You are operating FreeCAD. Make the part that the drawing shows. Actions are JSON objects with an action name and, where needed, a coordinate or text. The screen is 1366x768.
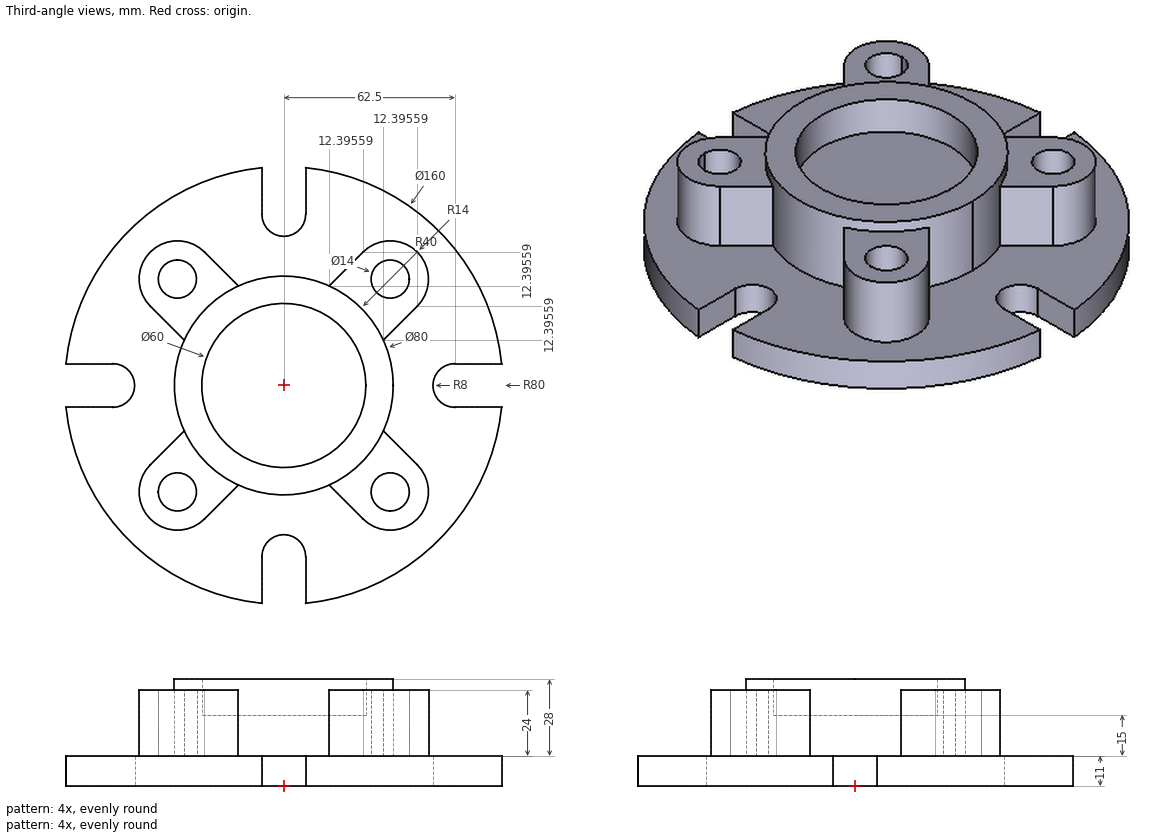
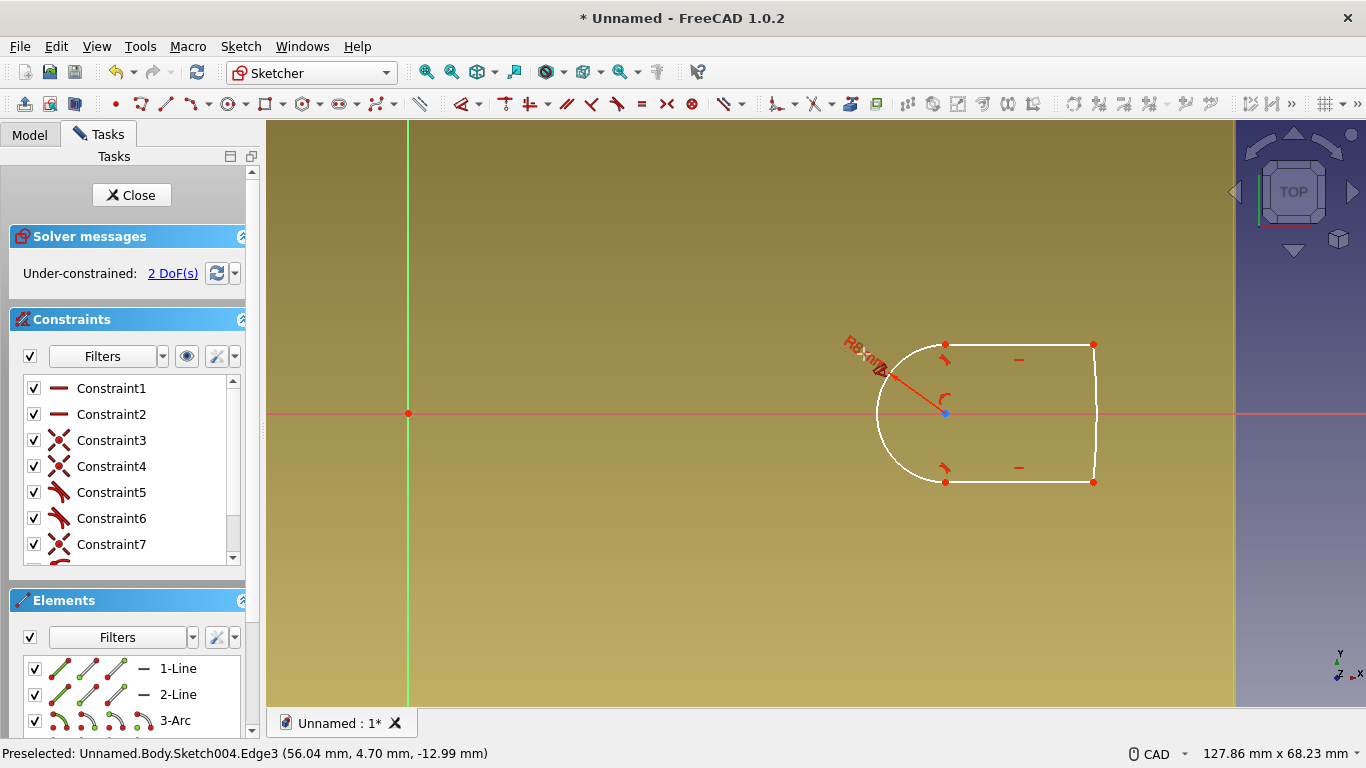
{"action": "left_click", "coordinate": [1096, 441]}
{"action": "left_click", "coordinate": [1128, 442]}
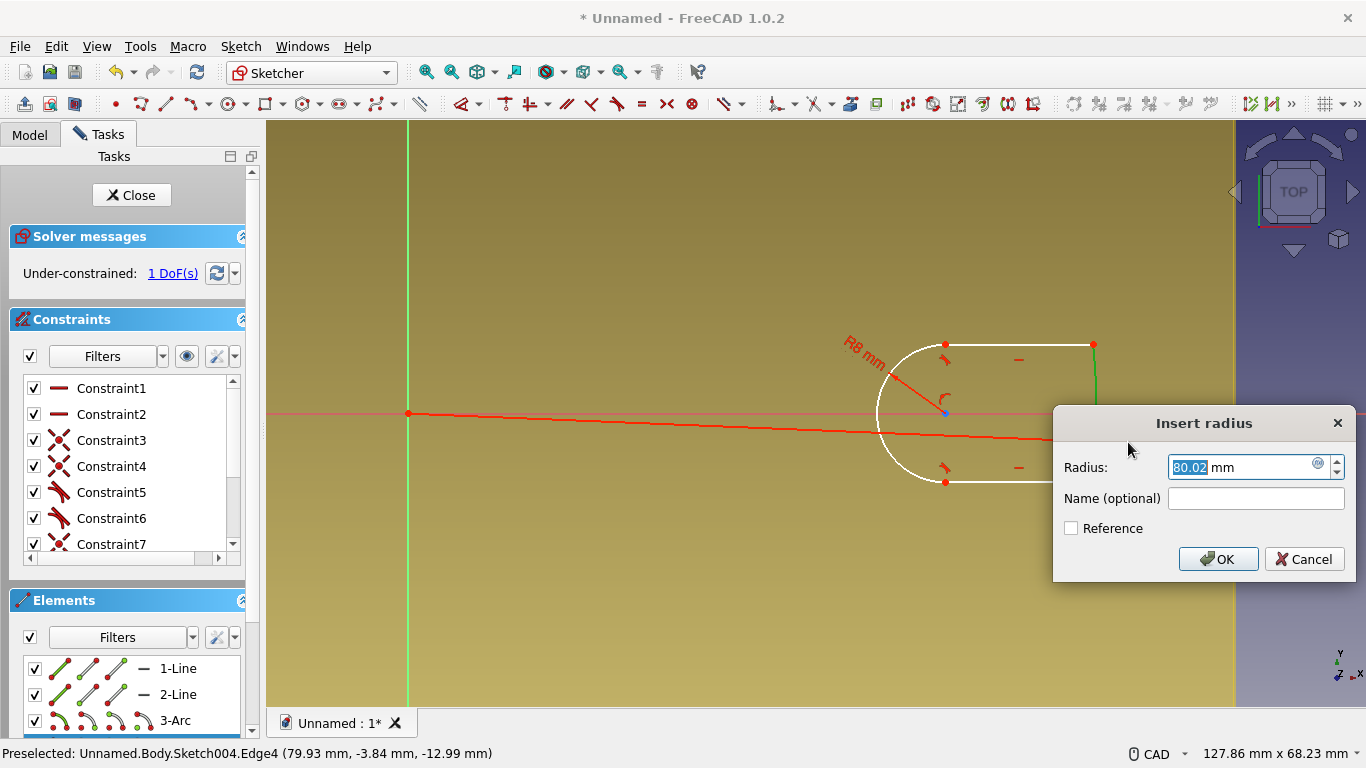
{"action": "type", "text": "80"}
{"action": "key", "text": "Return"}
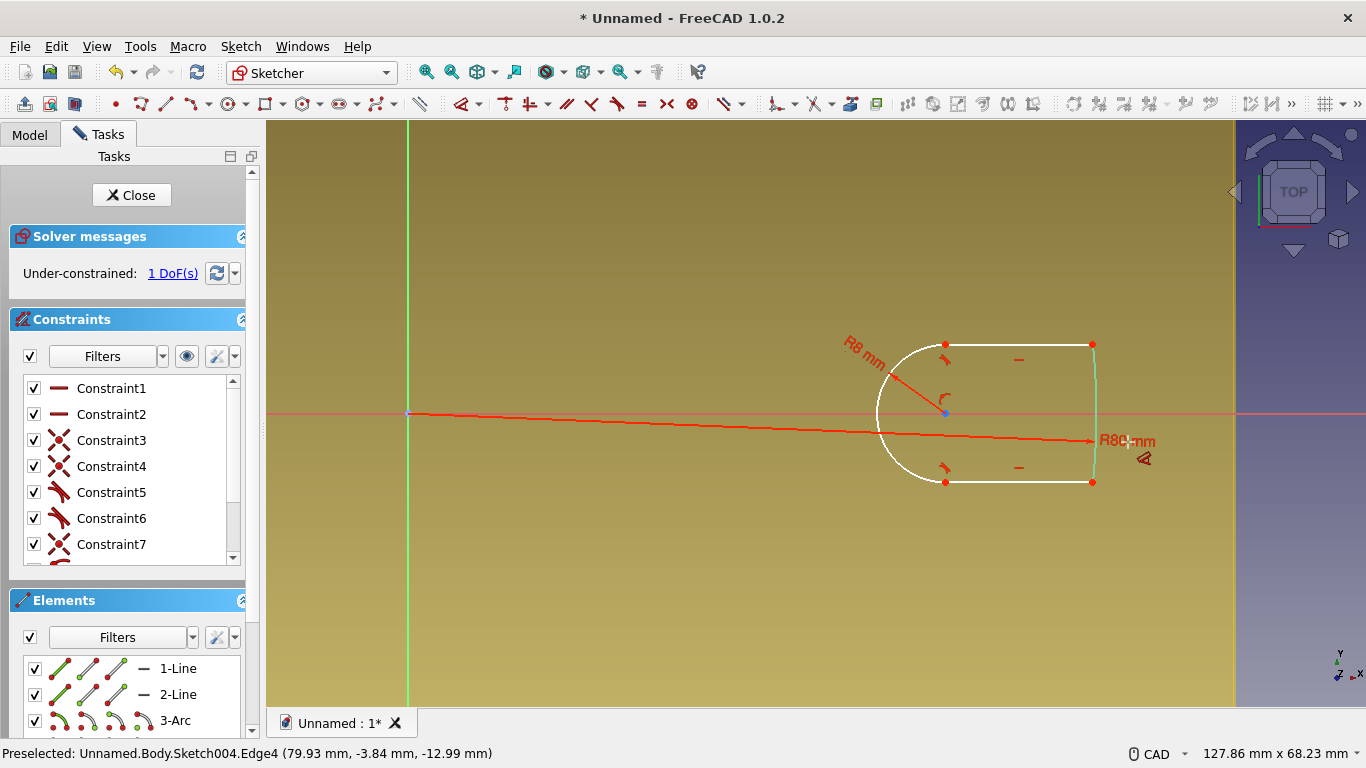
{"action": "left_click", "coordinate": [946, 345]}
{"action": "left_click", "coordinate": [677, 311]}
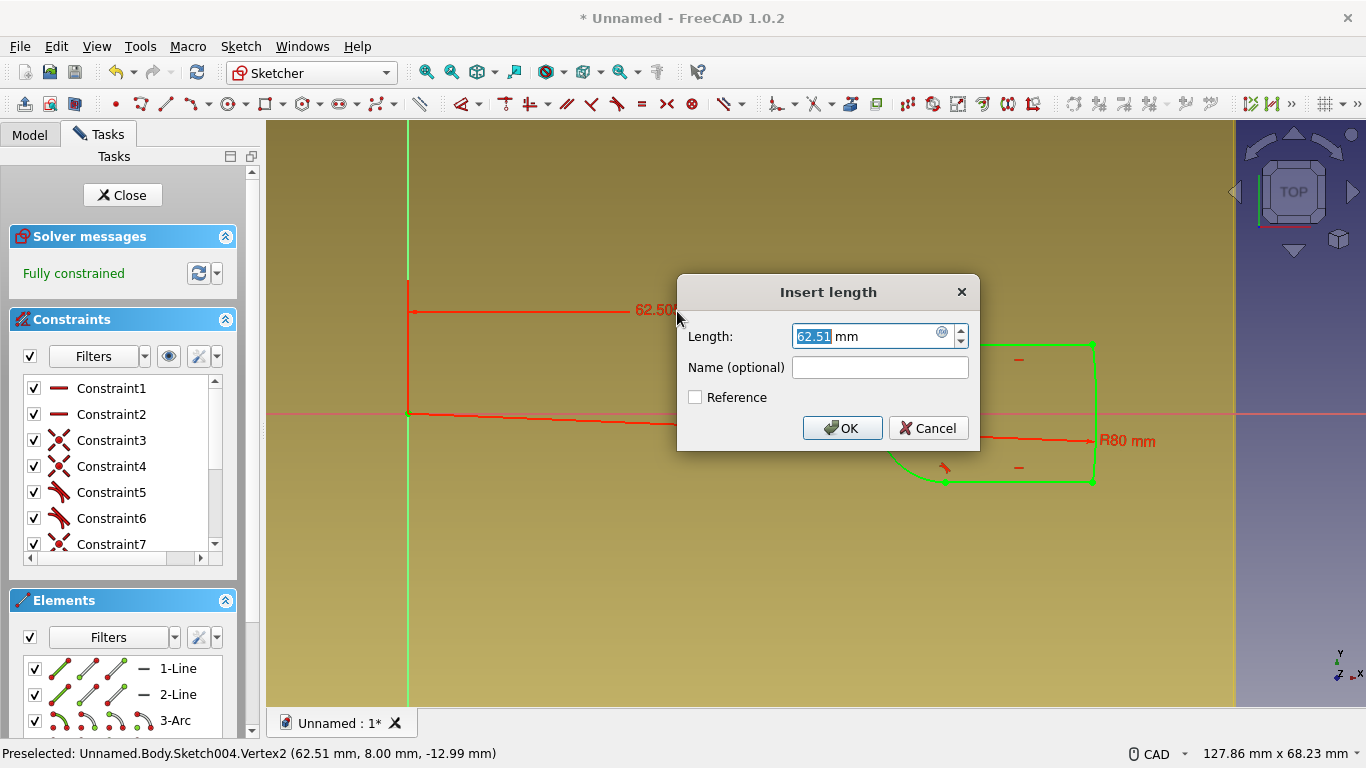
{"action": "type", "text": "62.5"}
{"action": "key", "text": "Return"}
{"action": "key", "text": "Escape"}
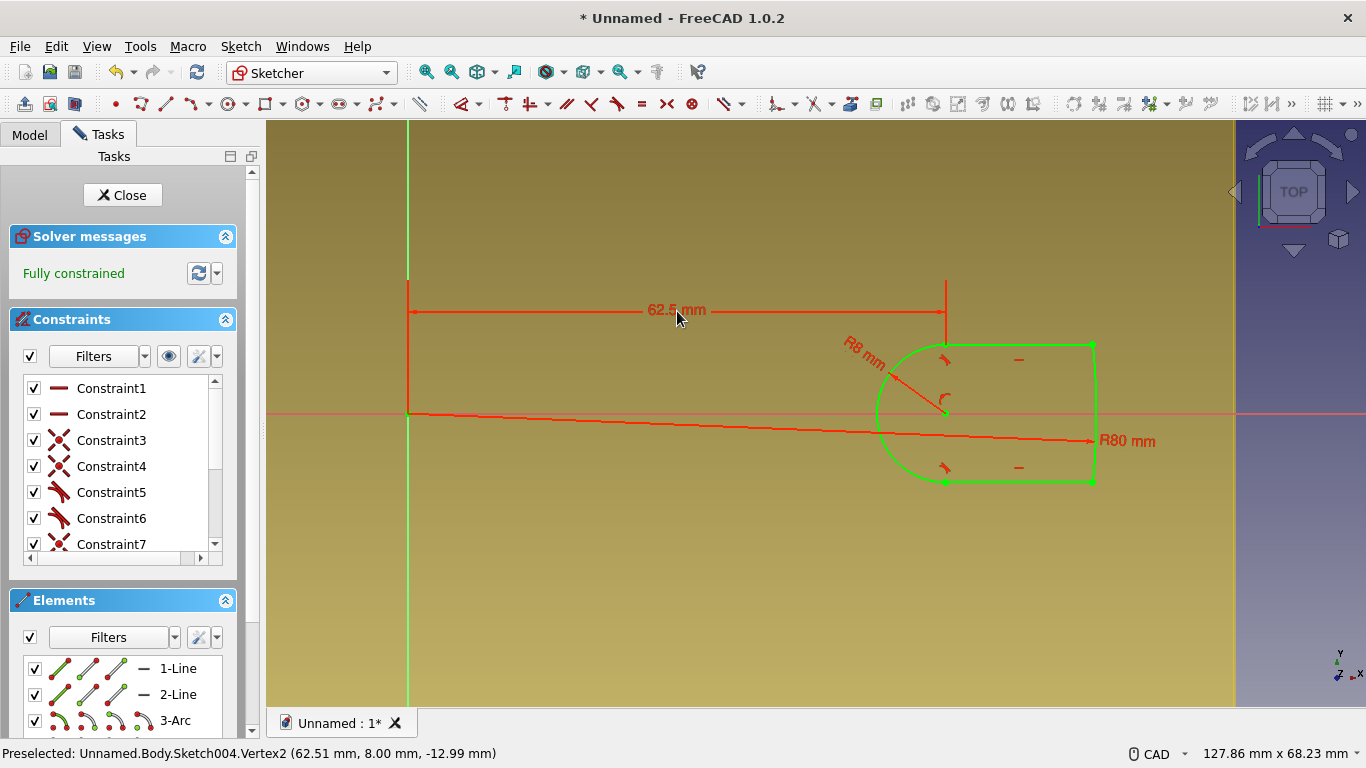
{"action": "left_click", "coordinate": [123, 195]}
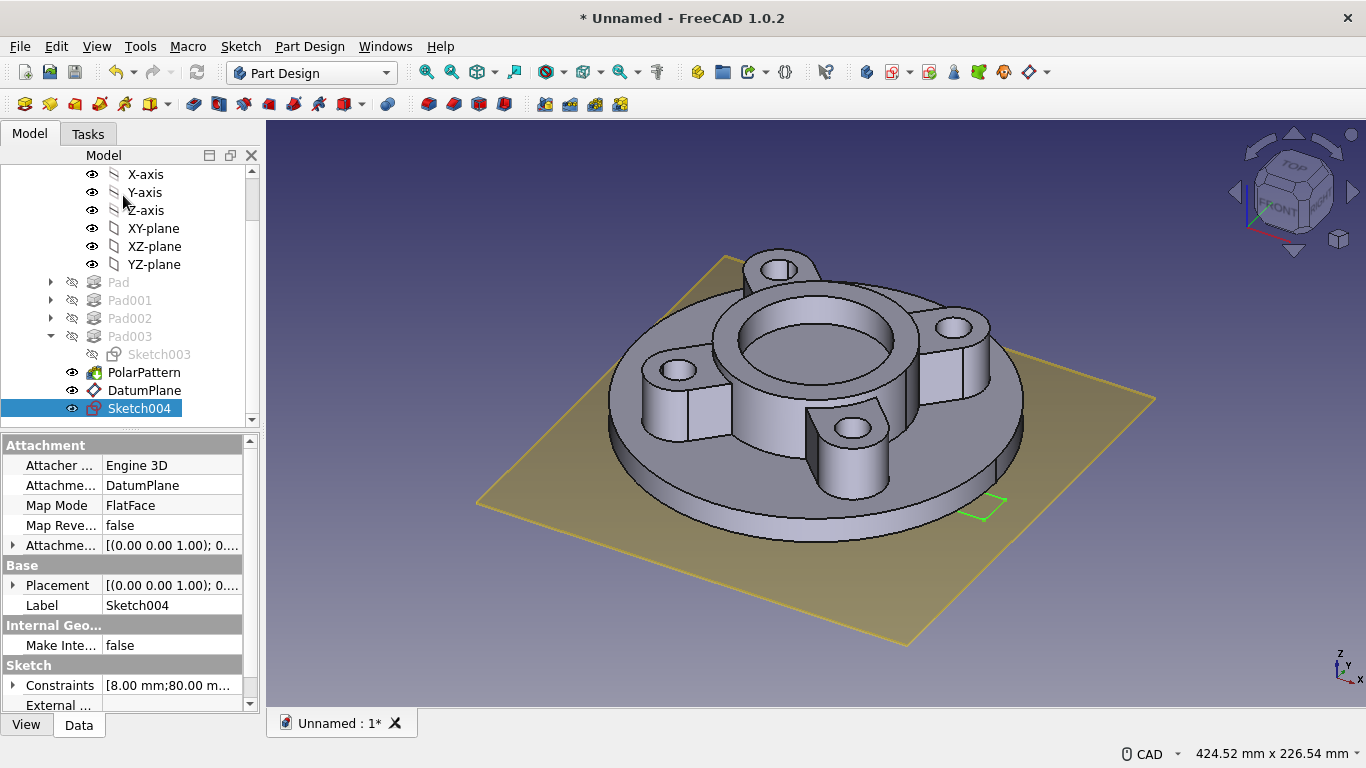
{"action": "left_click", "coordinate": [194, 104]}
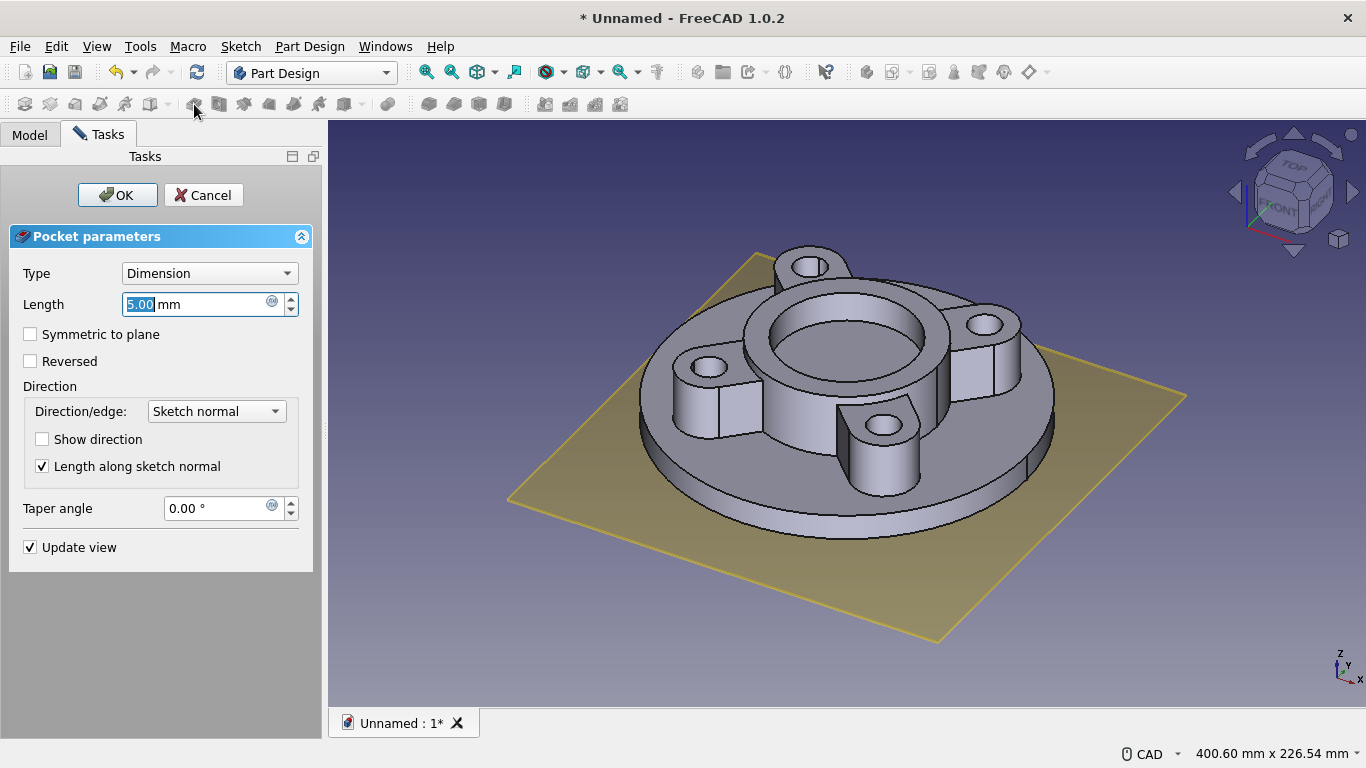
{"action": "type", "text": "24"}
{"action": "key", "text": "Tab"}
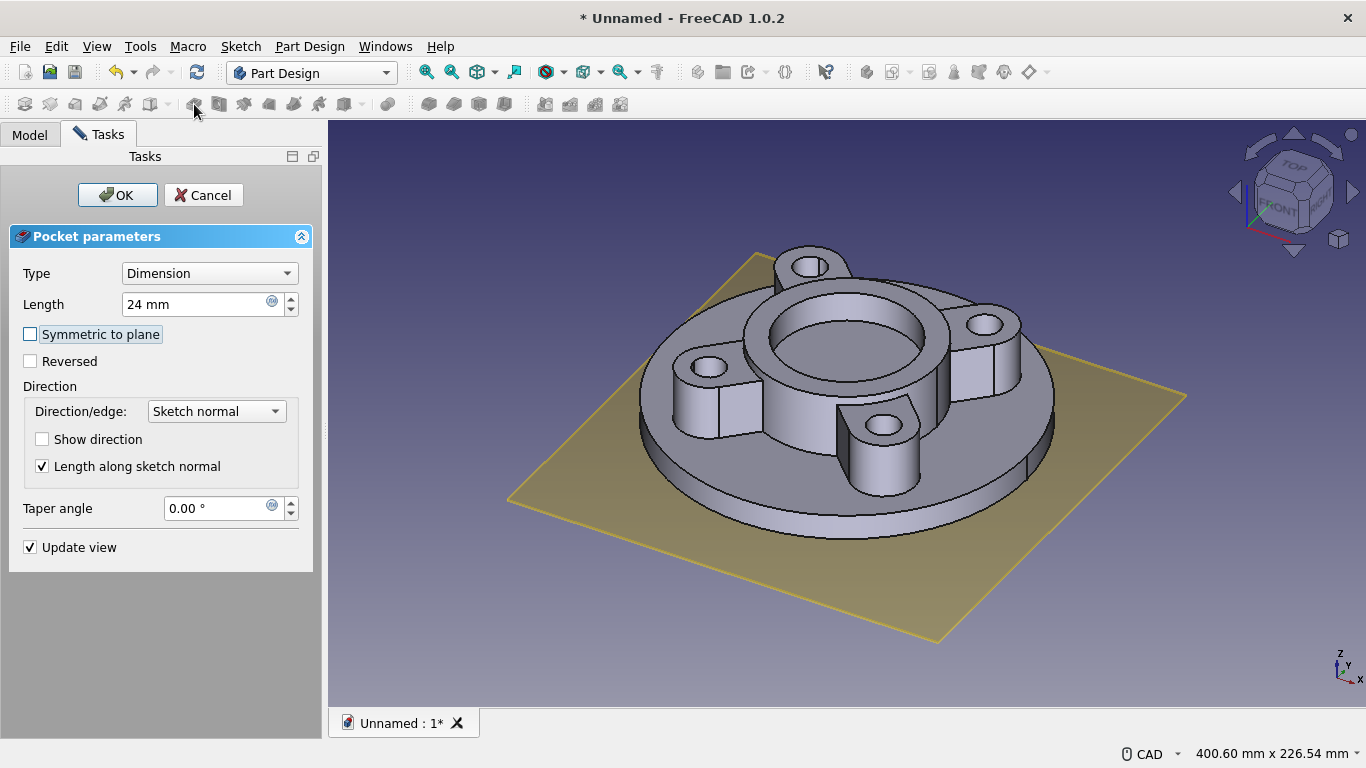
{"action": "left_click", "coordinate": [31, 361]}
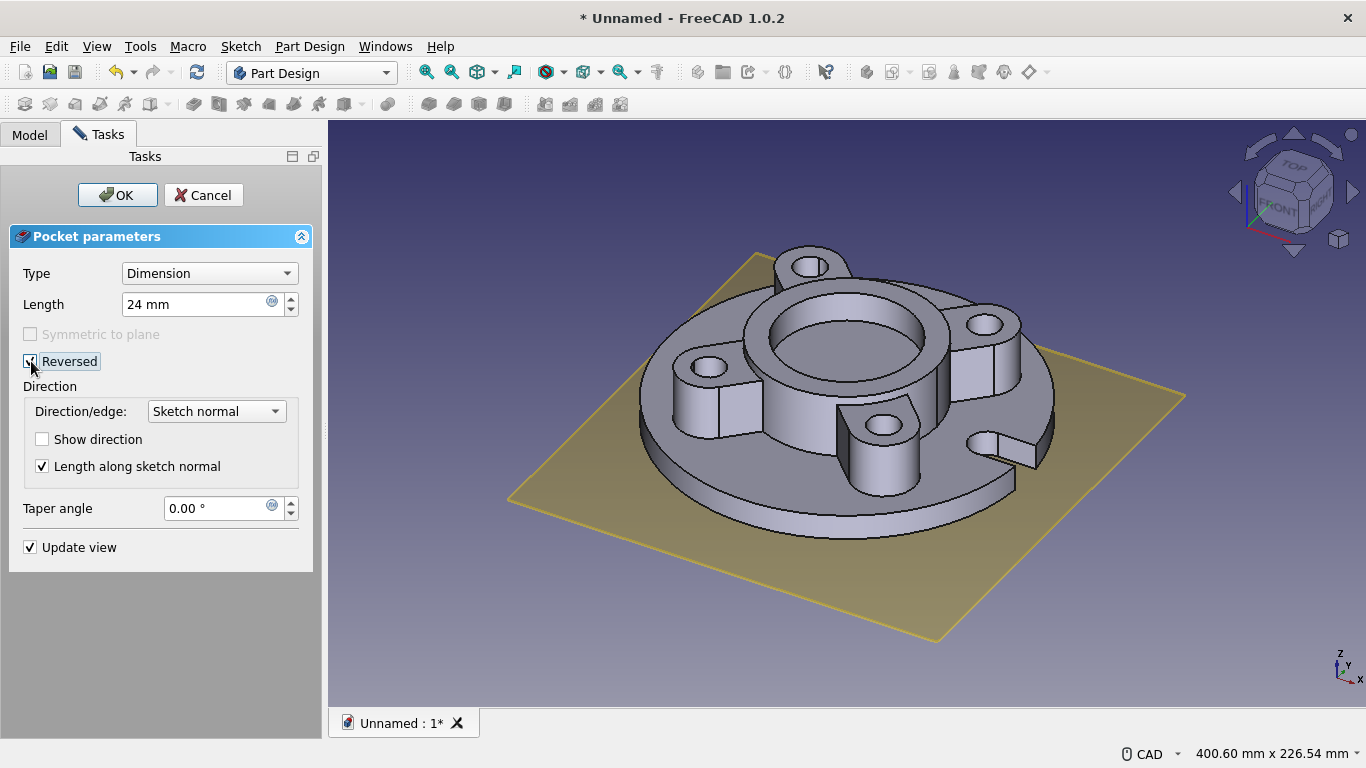
{"action": "left_click", "coordinate": [118, 195]}